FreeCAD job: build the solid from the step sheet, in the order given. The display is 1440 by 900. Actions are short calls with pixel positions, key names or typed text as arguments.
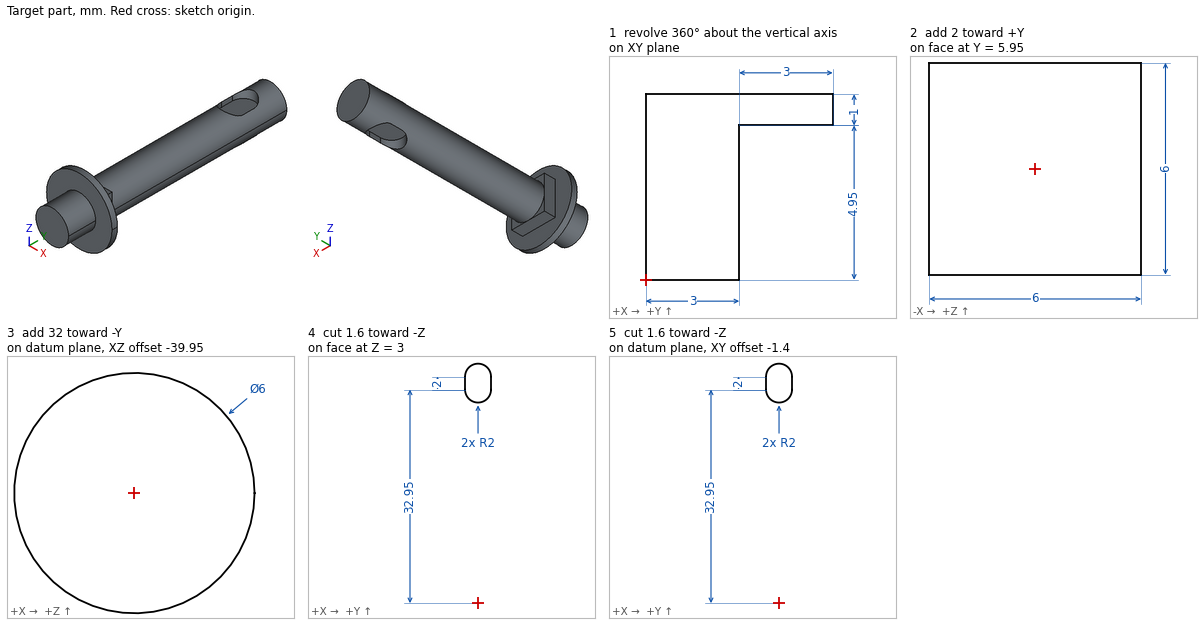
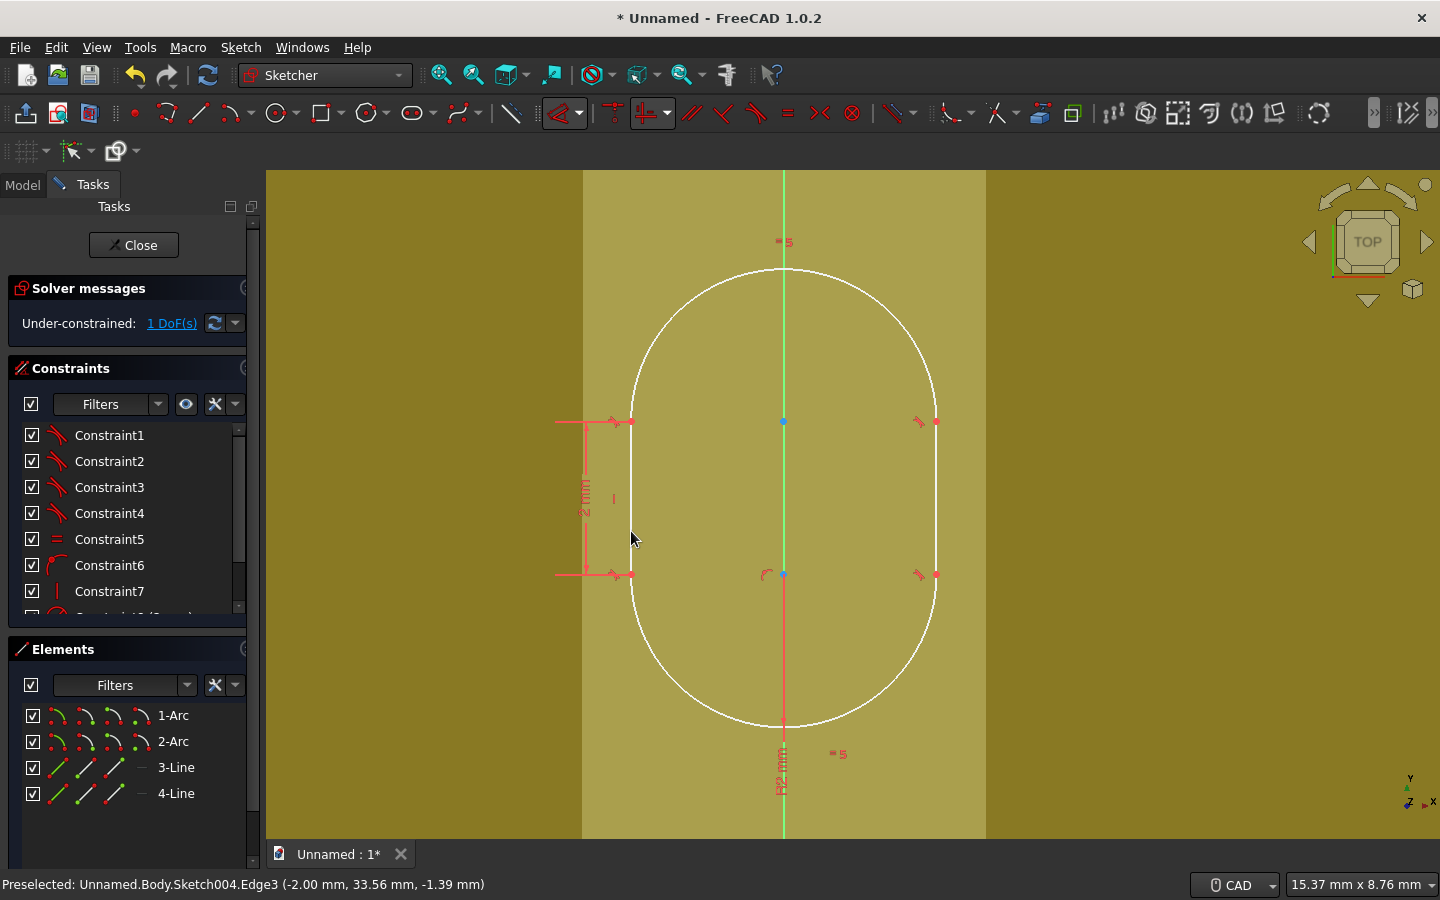
click(631, 575)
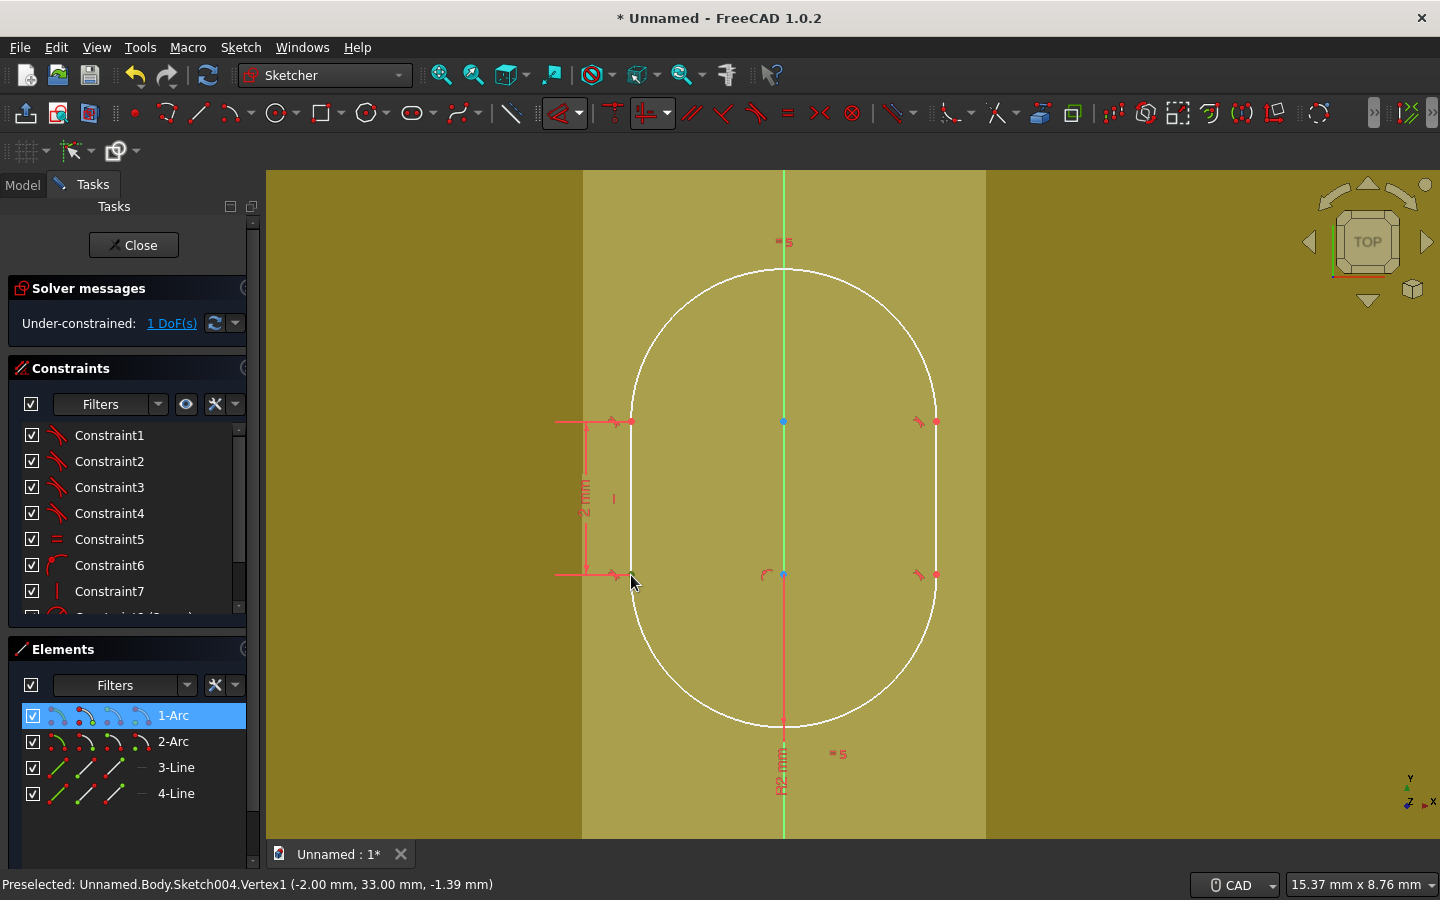
click(582, 114)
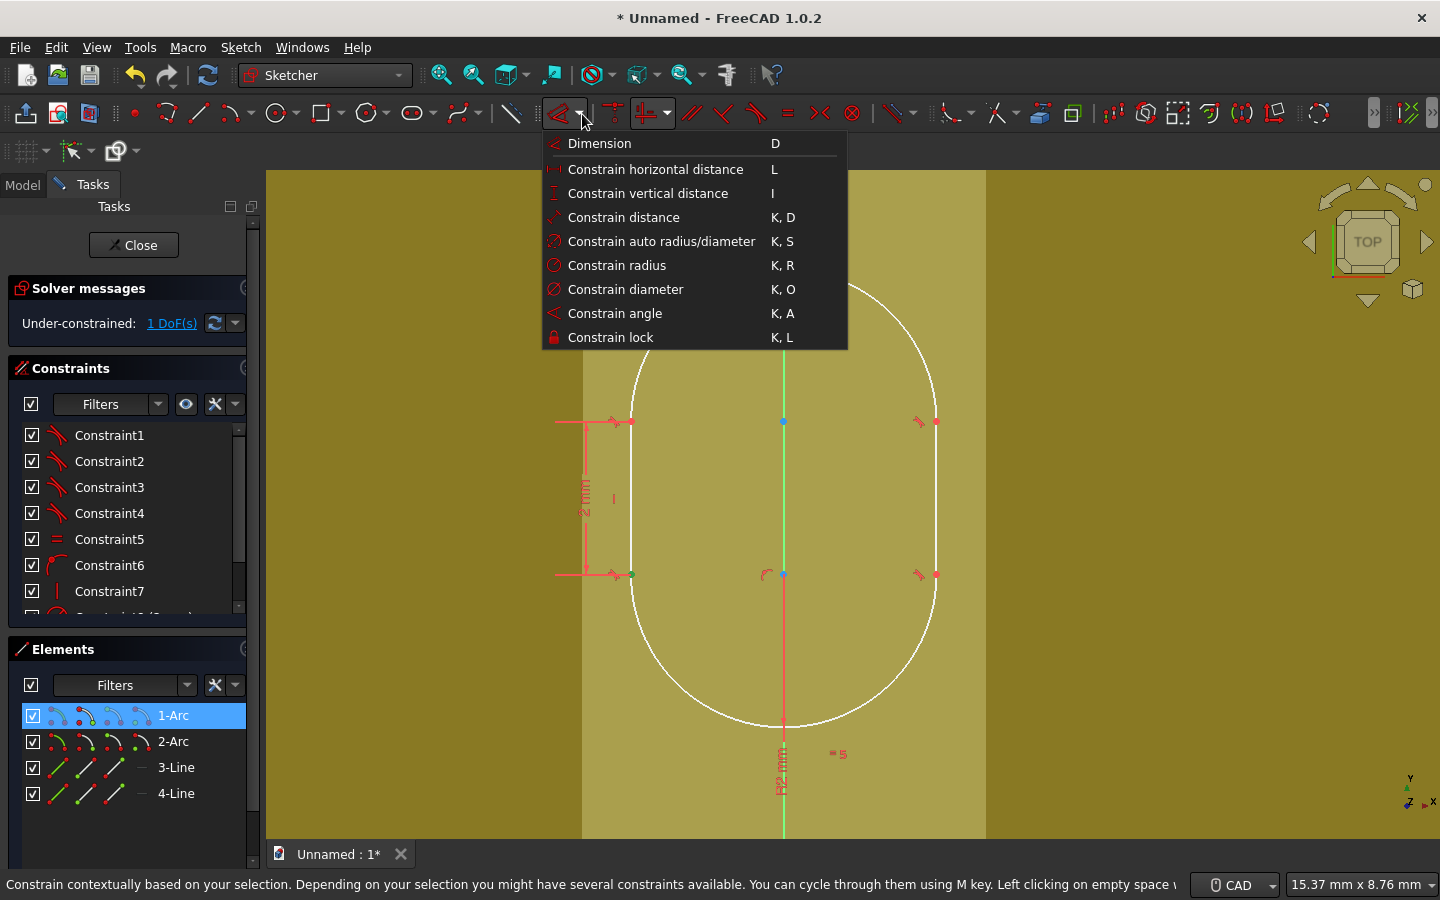
click(695, 193)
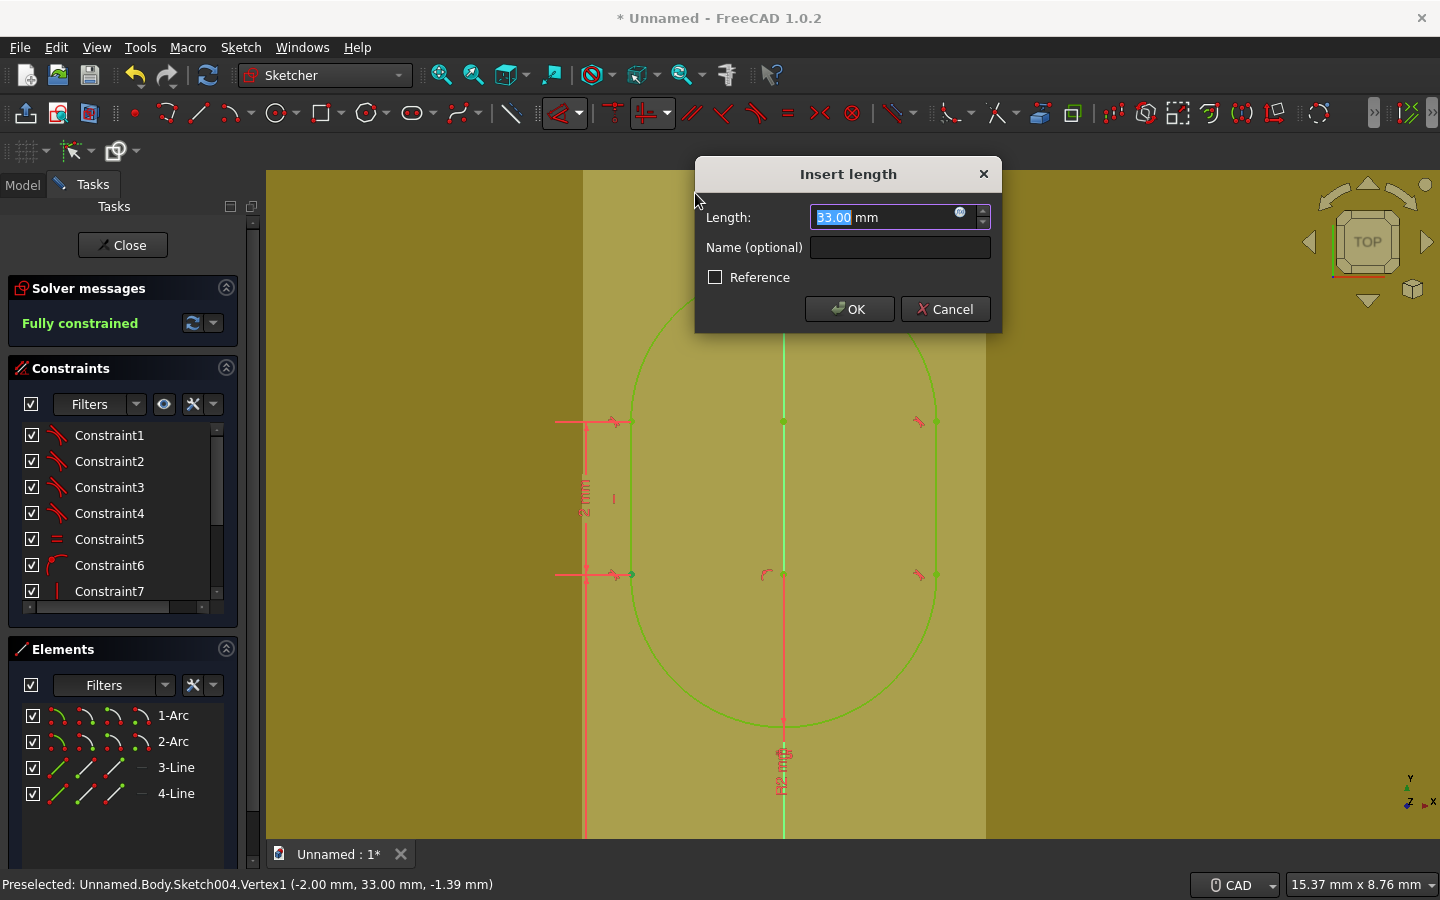
text(32.95)
key(Return)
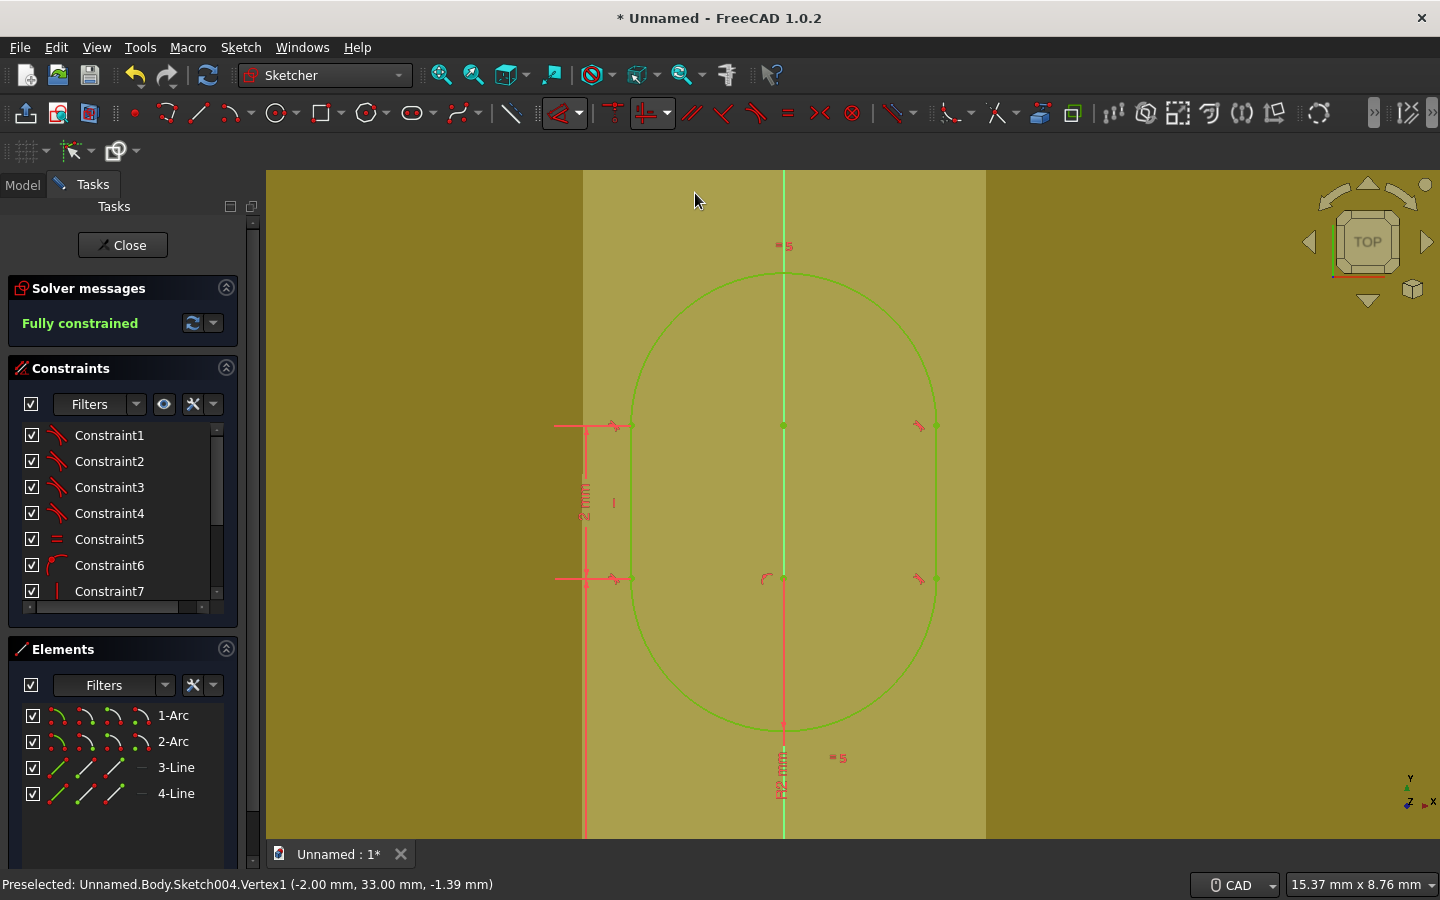
click(123, 245)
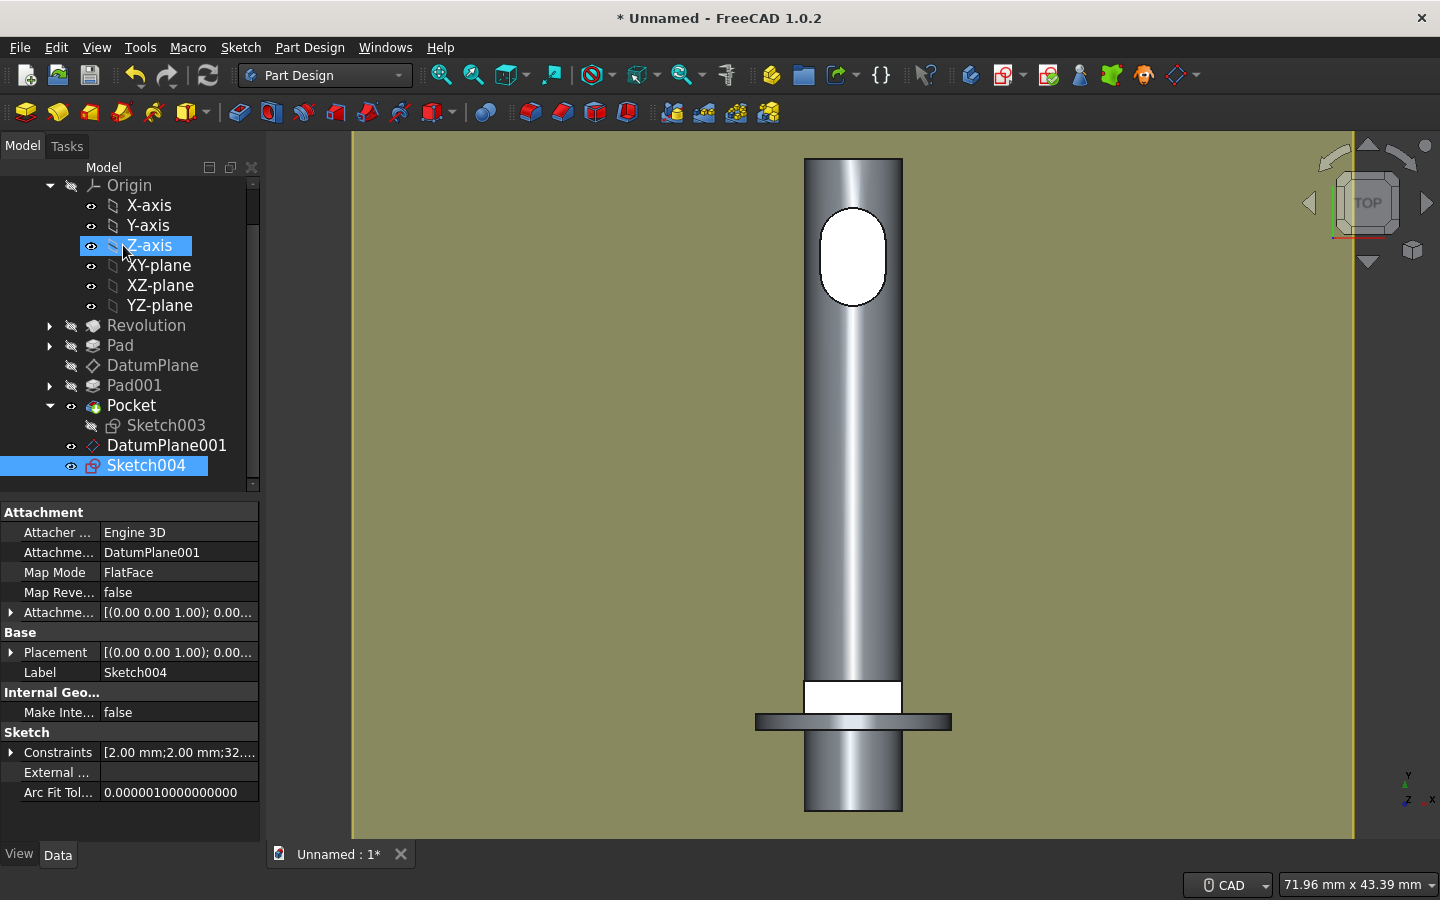
click(240, 112)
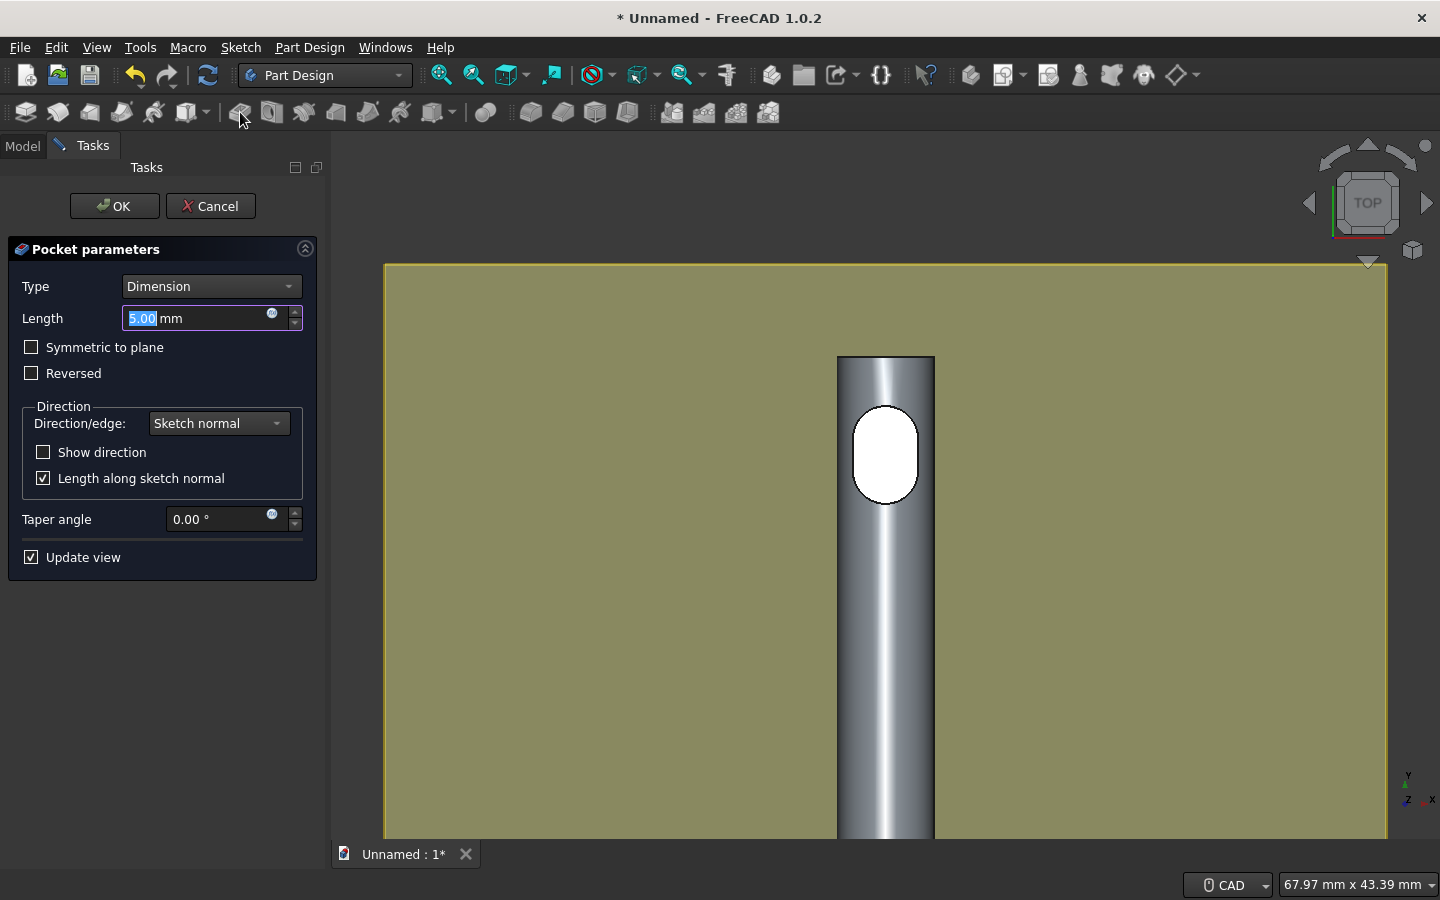
text(1.6)
key(Tab)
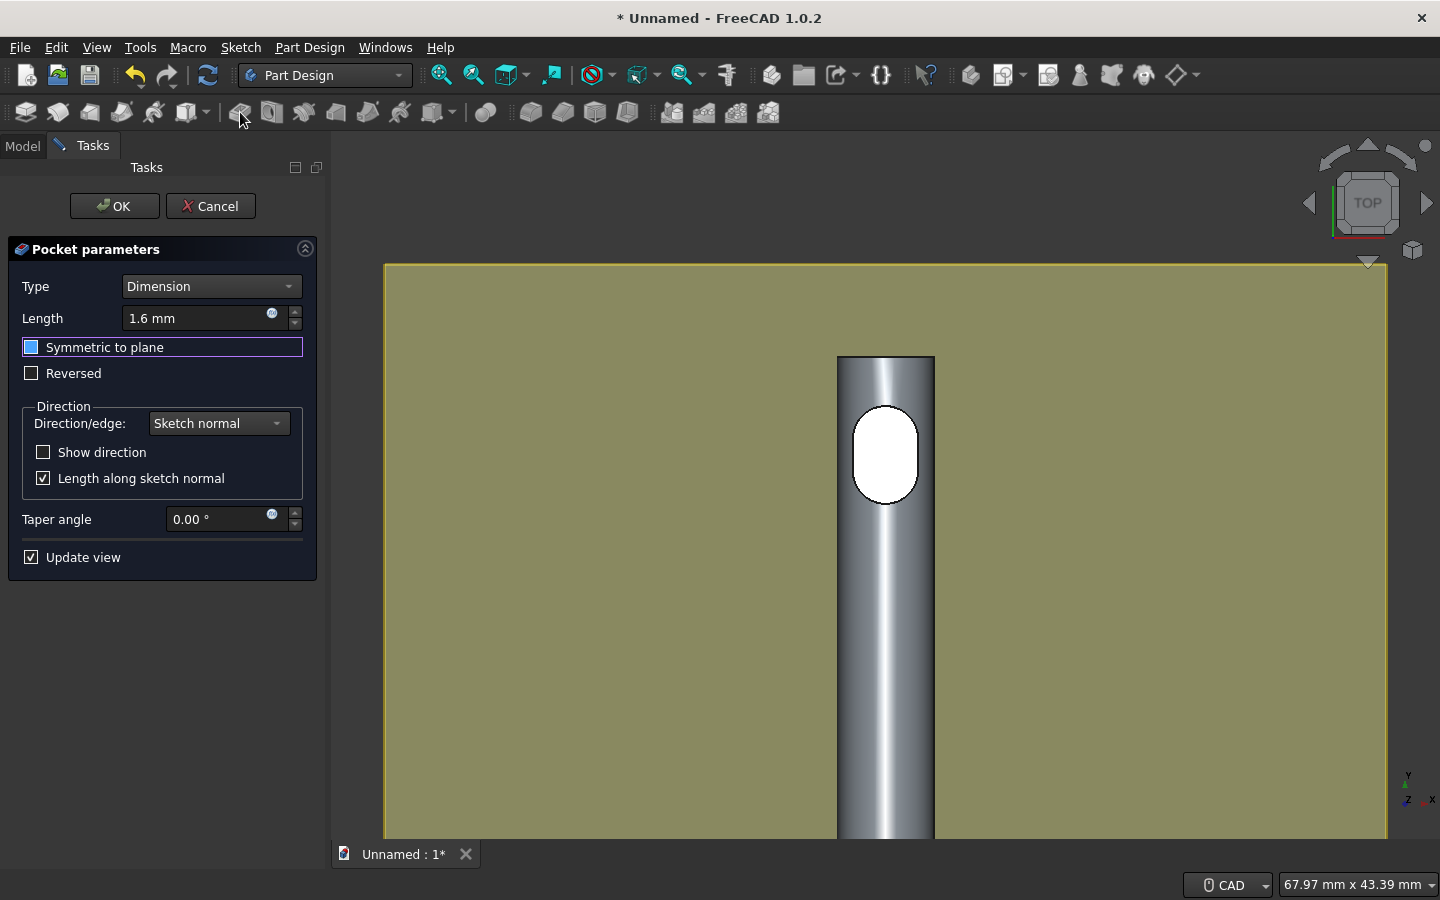
click(115, 206)